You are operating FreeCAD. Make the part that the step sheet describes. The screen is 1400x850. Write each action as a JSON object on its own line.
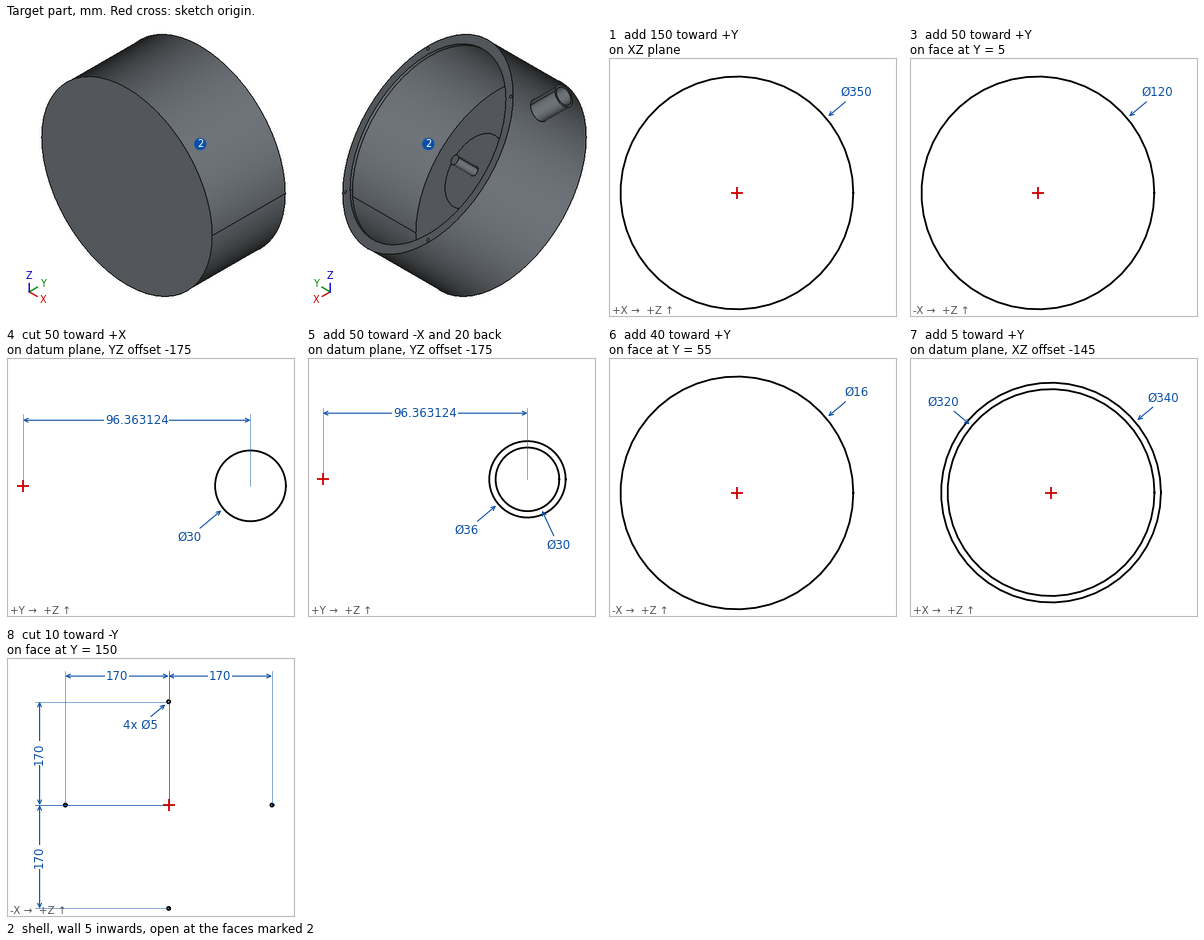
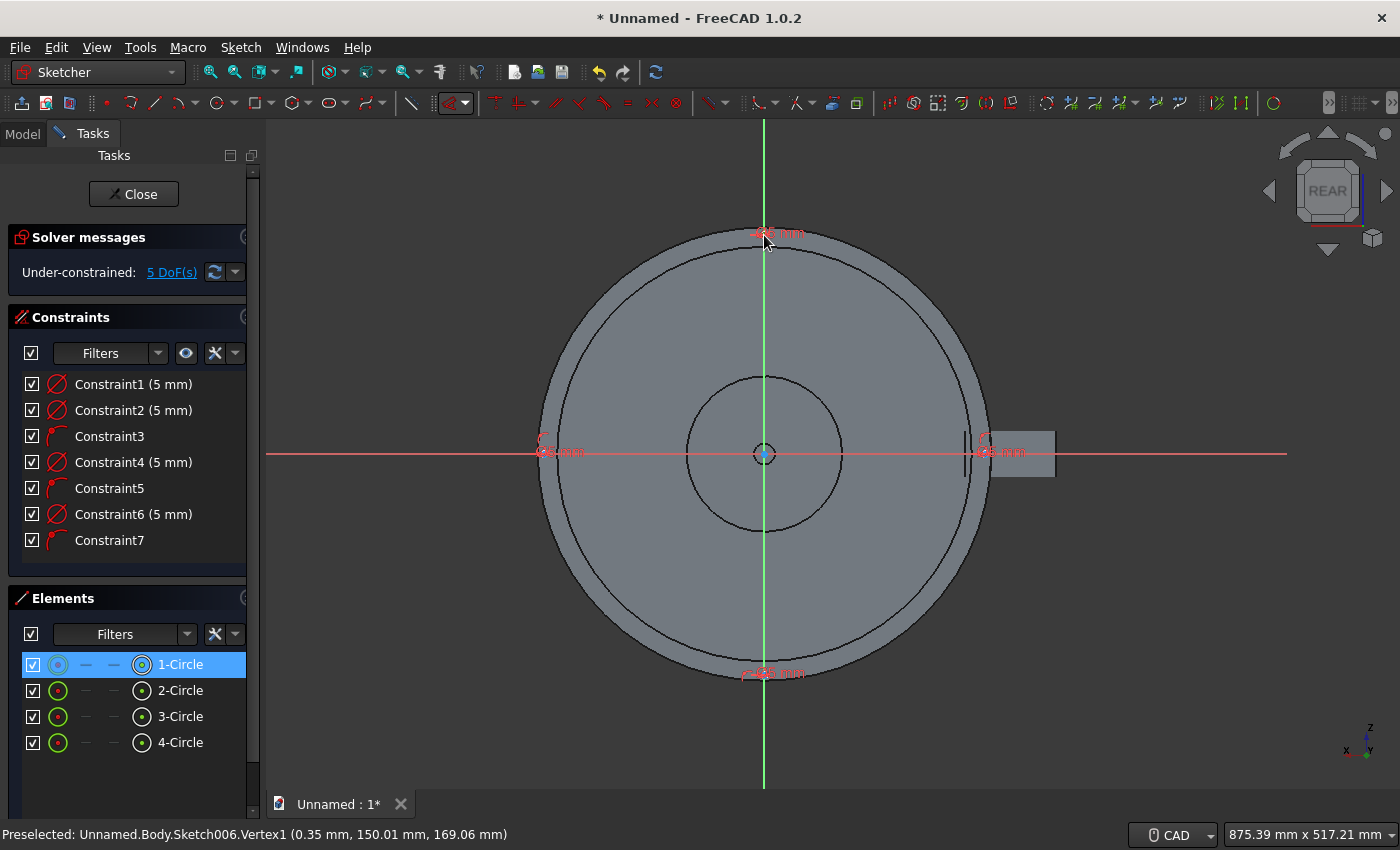
{"action": "left_click", "coordinate": [764, 717]}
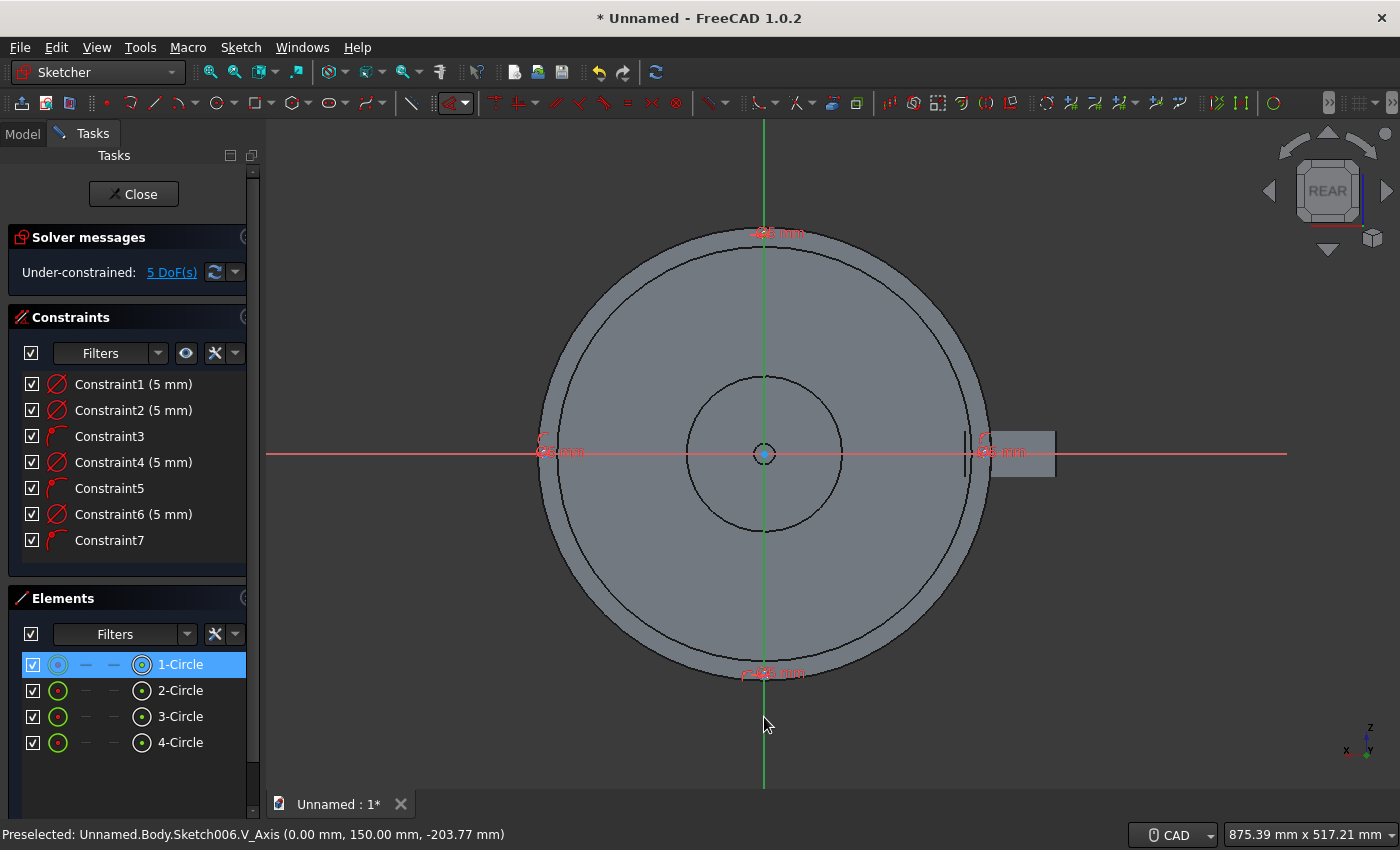
{"action": "left_click", "coordinate": [496, 104]}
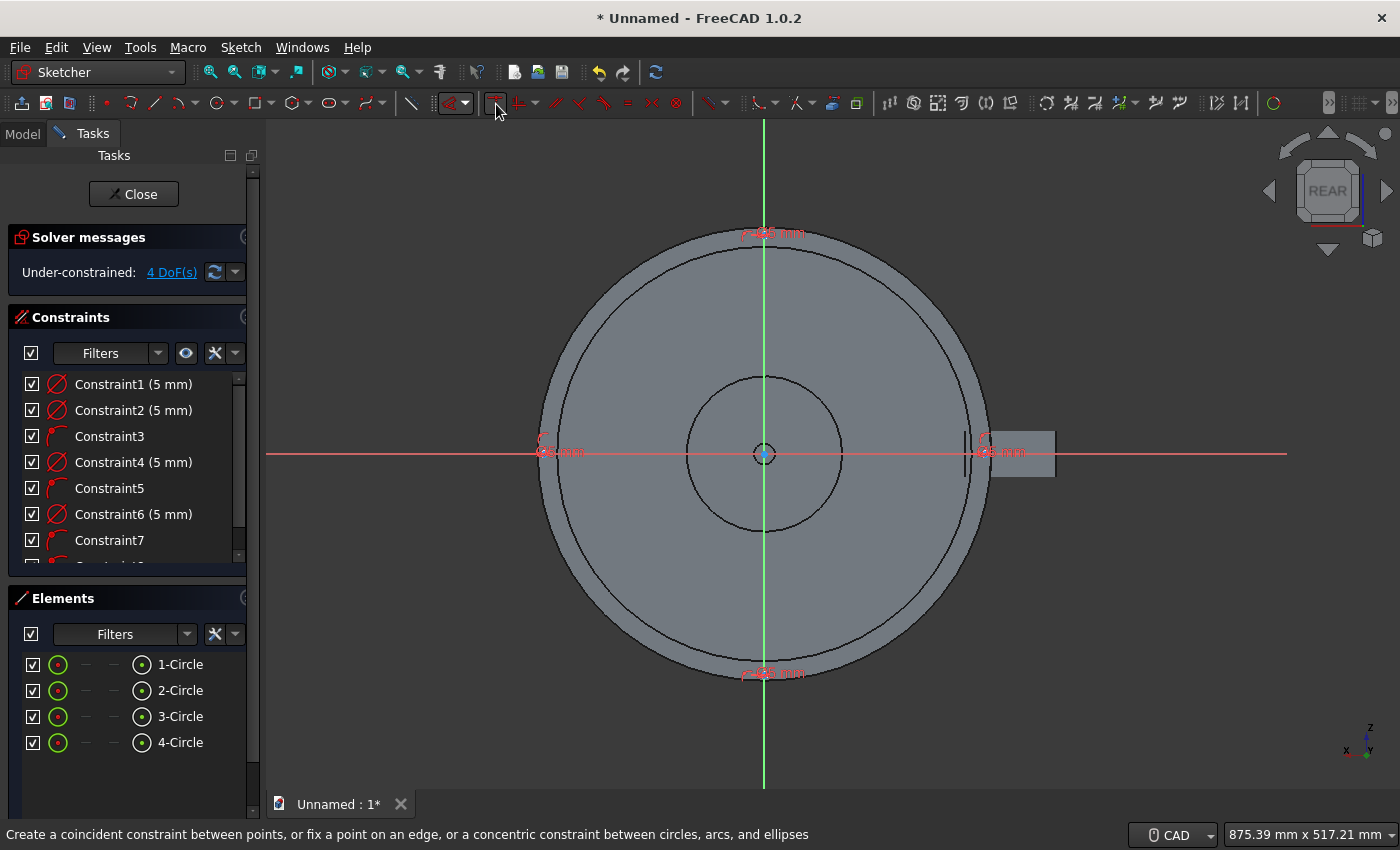
{"action": "left_click", "coordinate": [764, 235]}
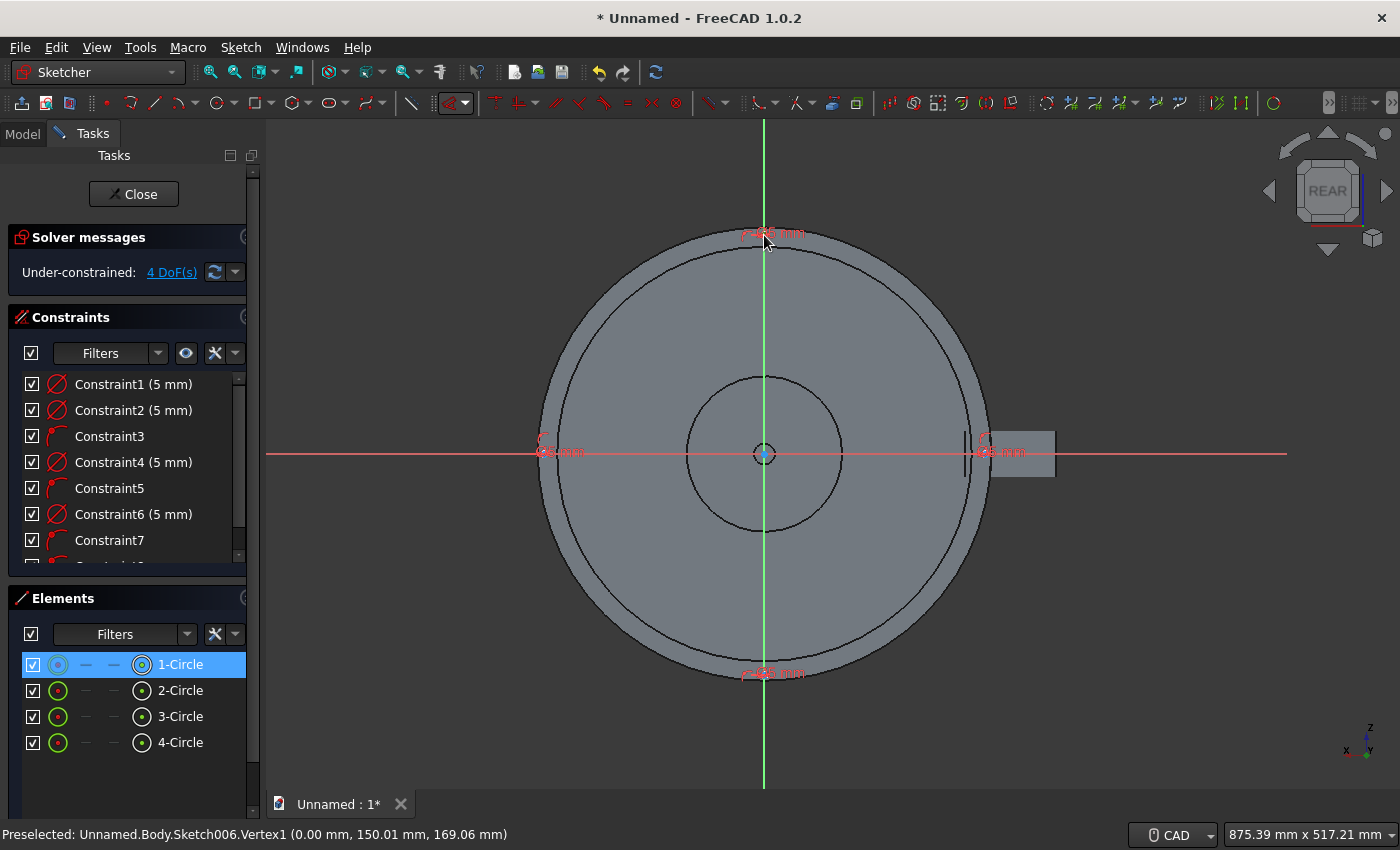
{"action": "key", "text": "i"}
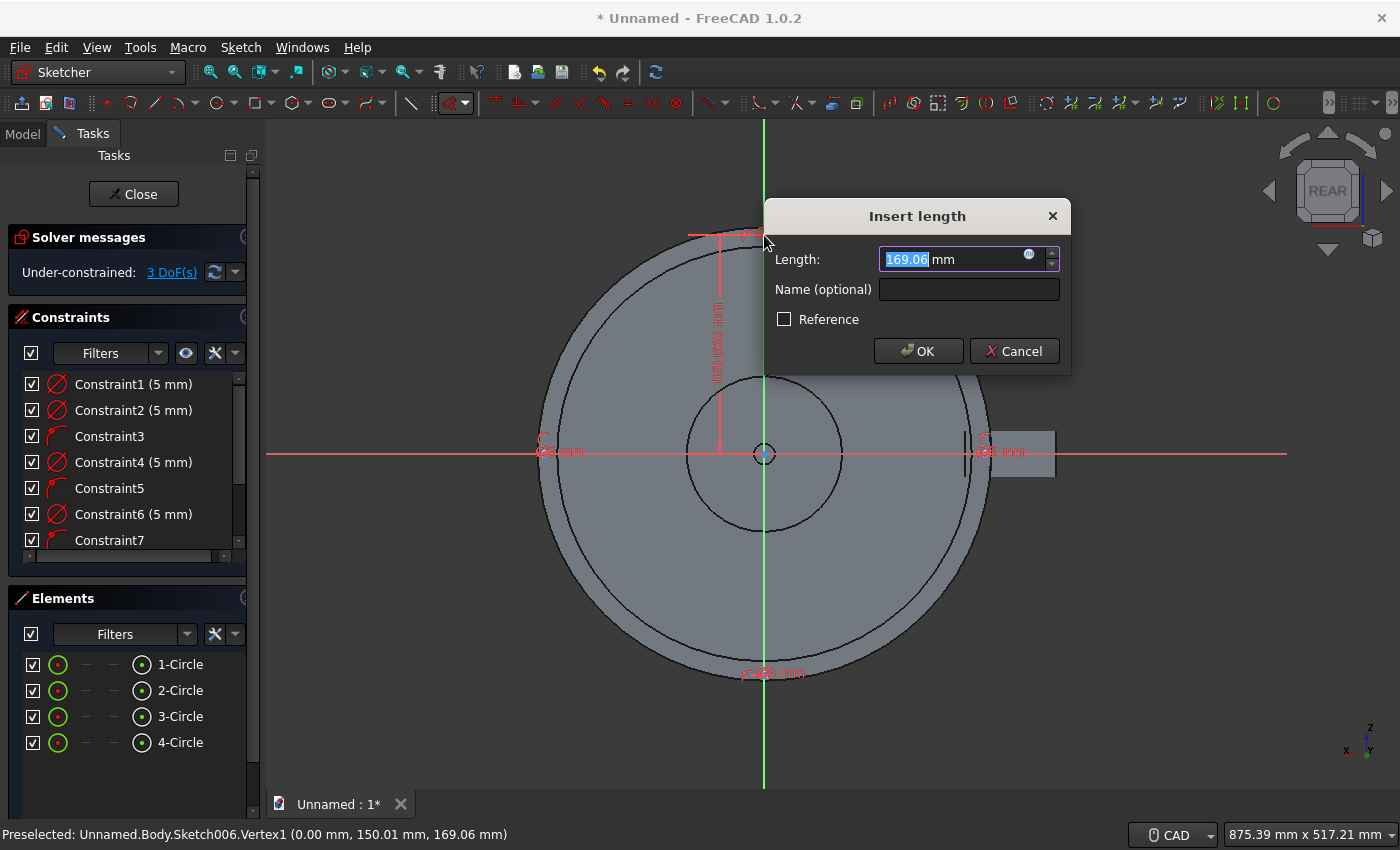
{"action": "type", "text": "170"}
{"action": "key", "text": "Return"}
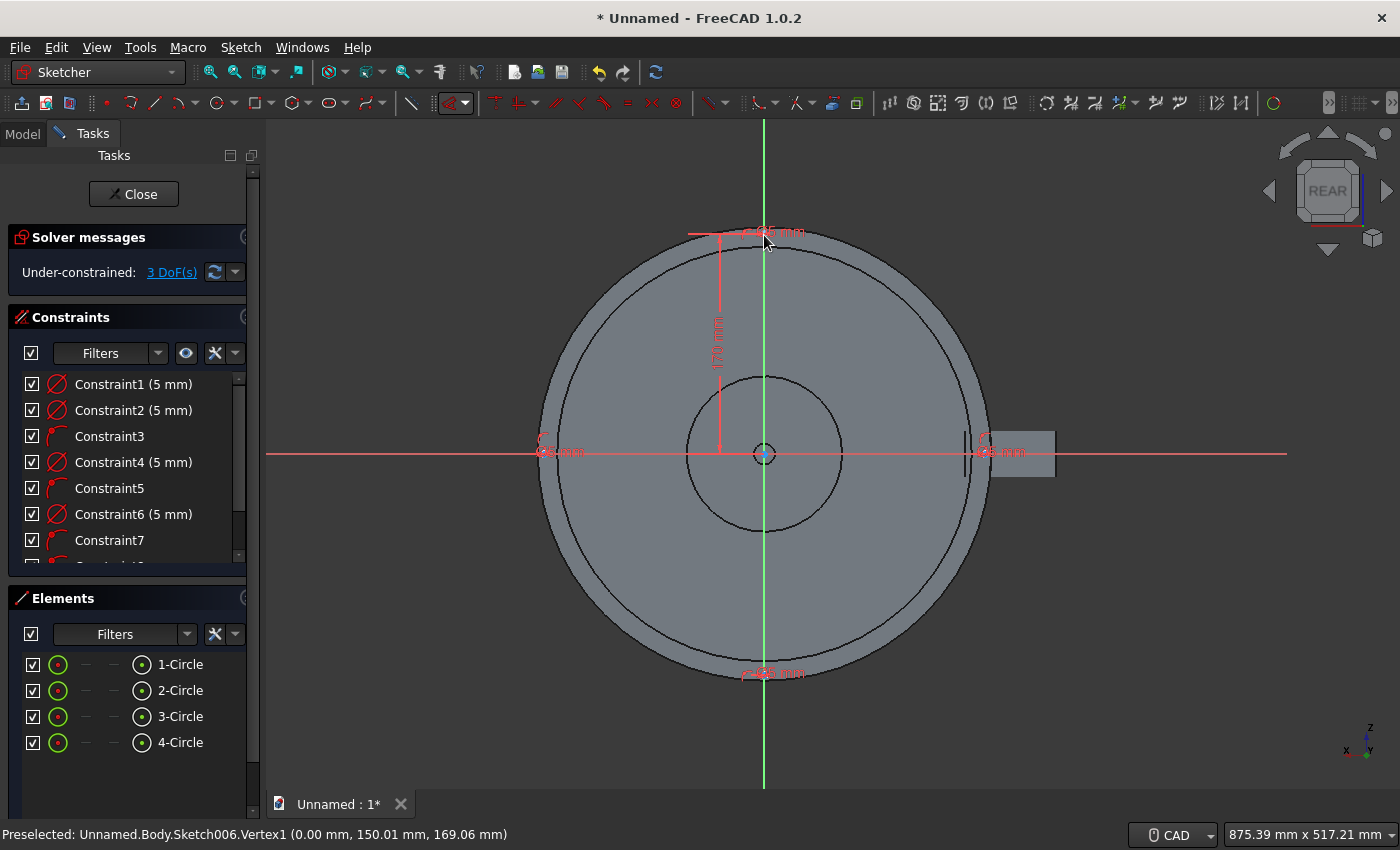
{"action": "left_click", "coordinate": [985, 454]}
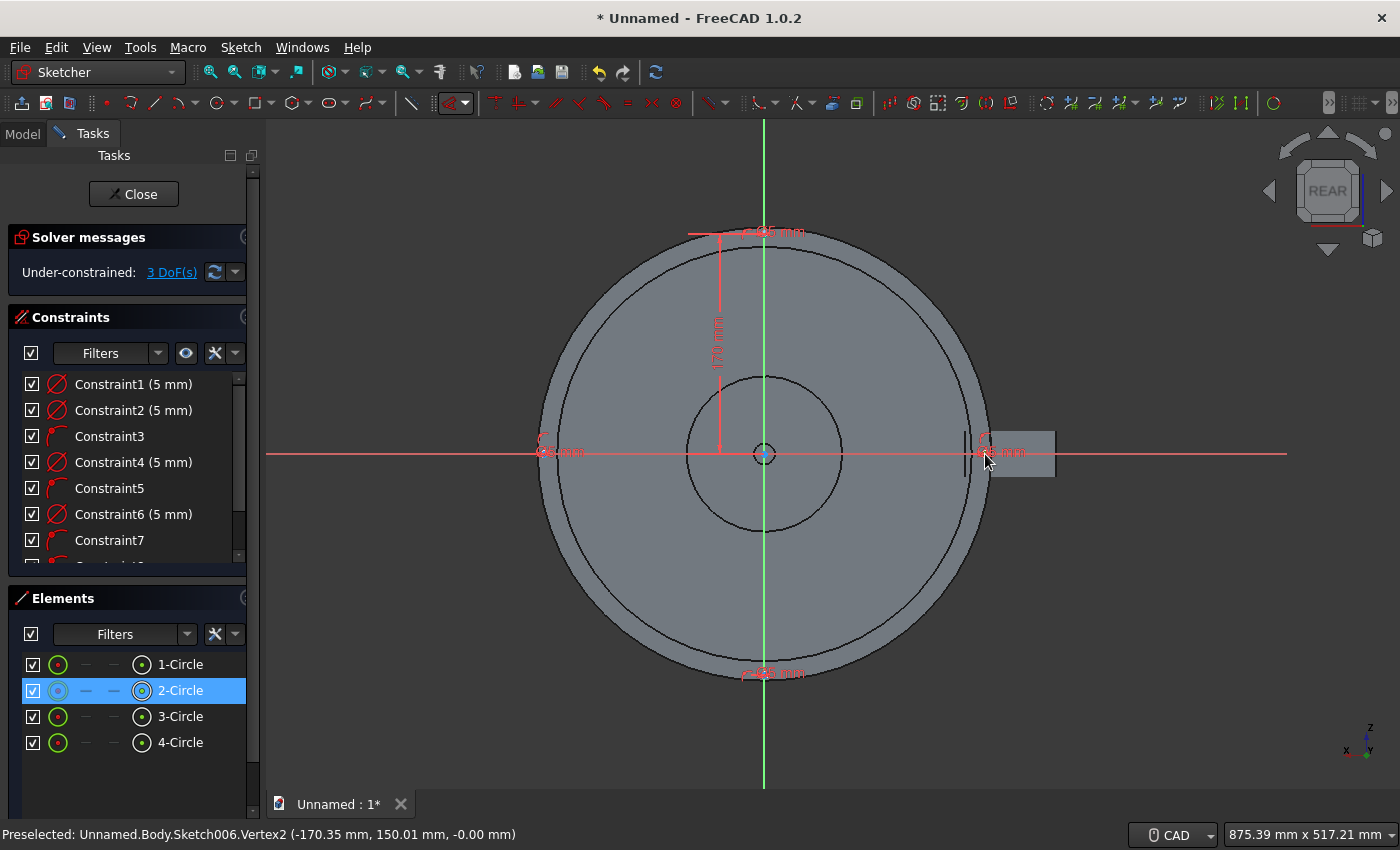
{"action": "left_click", "coordinate": [468, 104]}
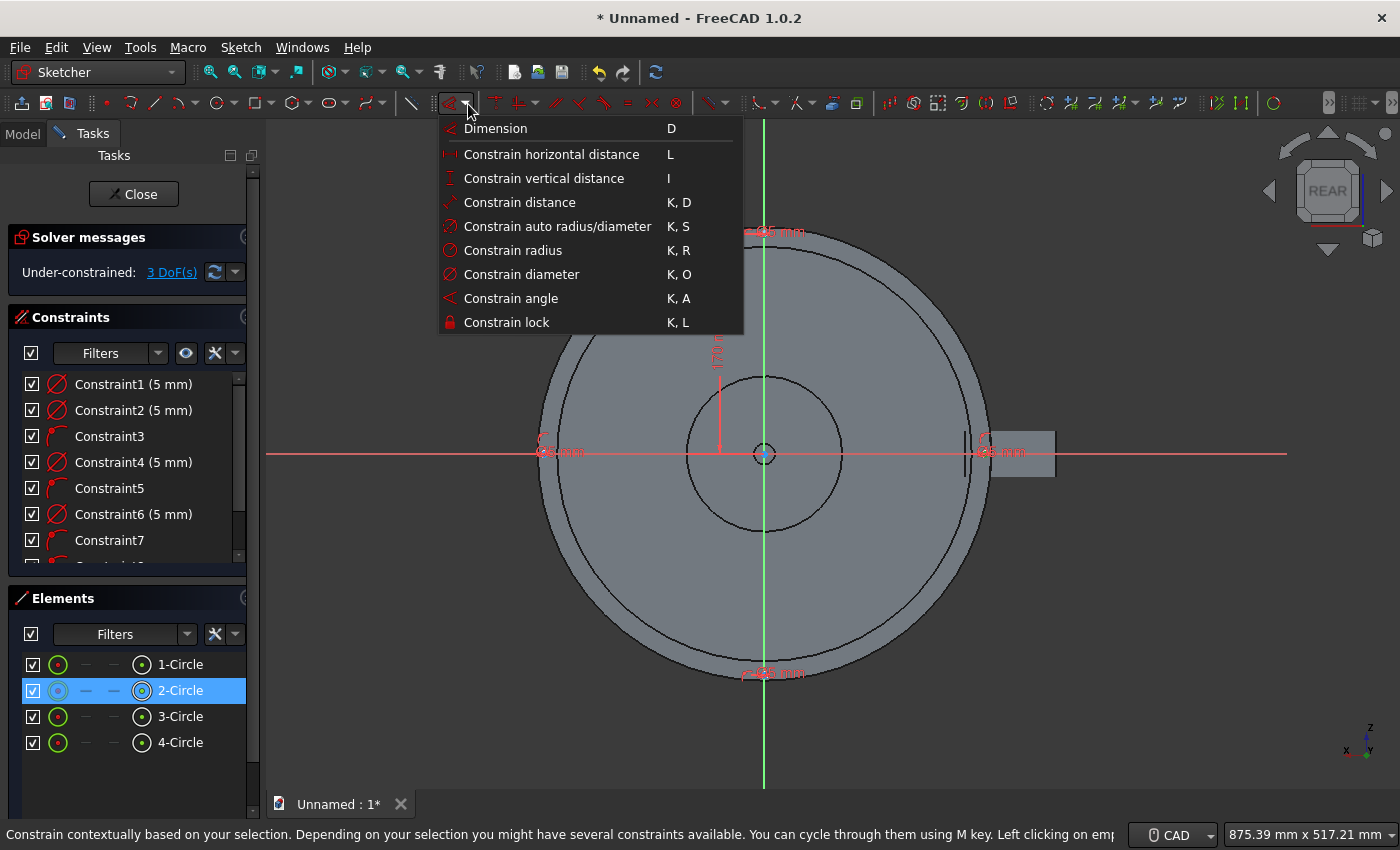
{"action": "left_click", "coordinate": [591, 154]}